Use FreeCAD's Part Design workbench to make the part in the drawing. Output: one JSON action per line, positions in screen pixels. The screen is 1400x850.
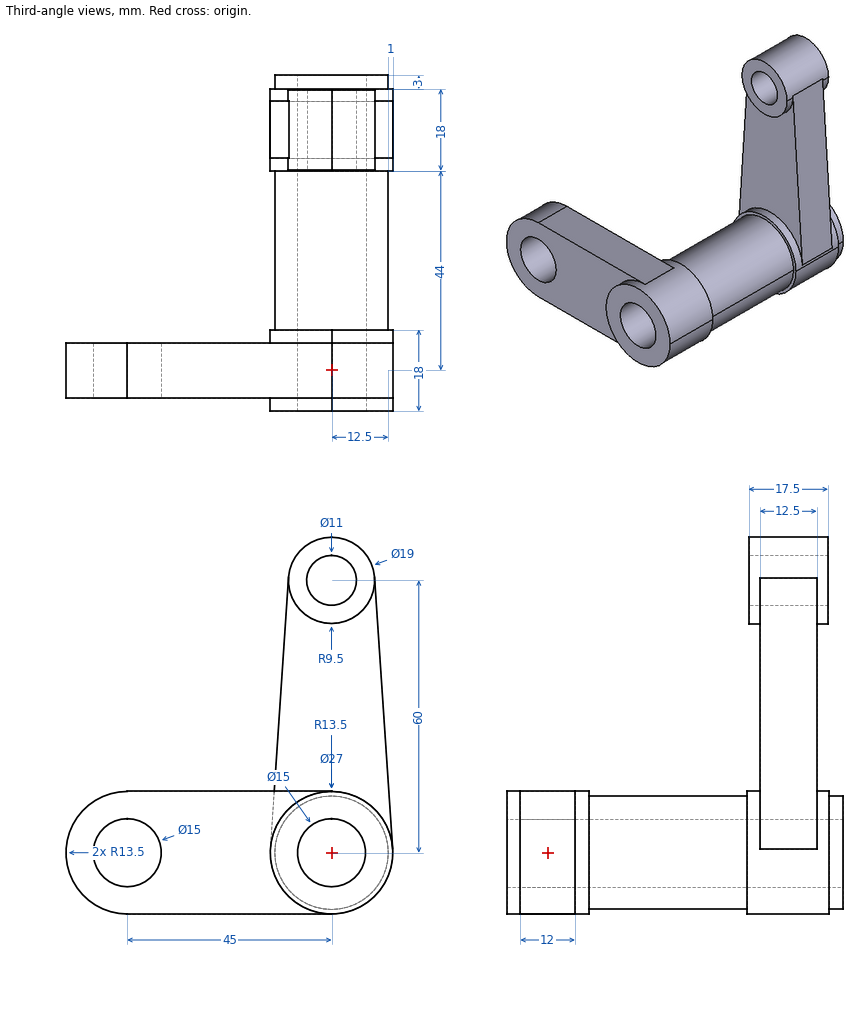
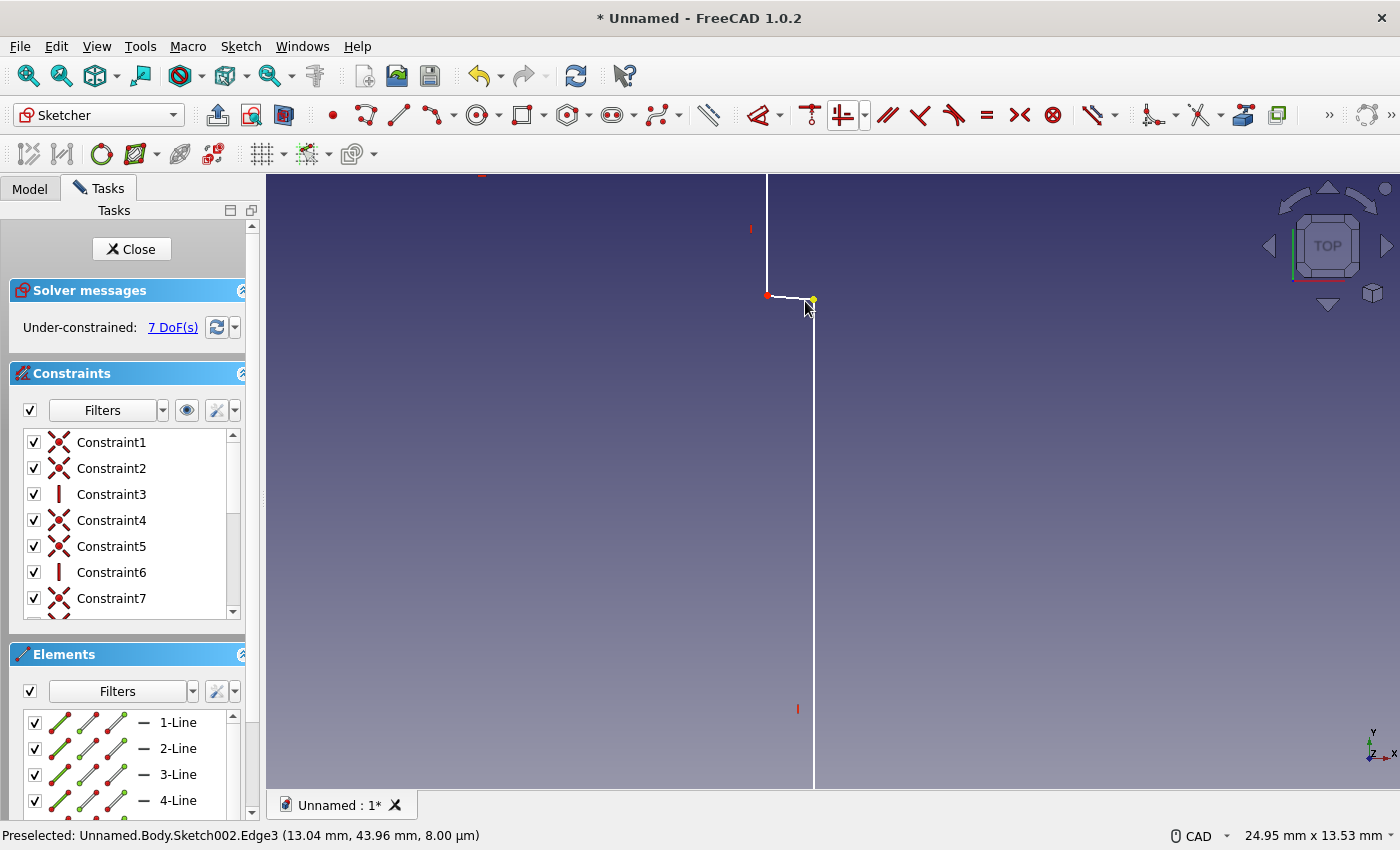
{"action": "left_click", "coordinate": [800, 299]}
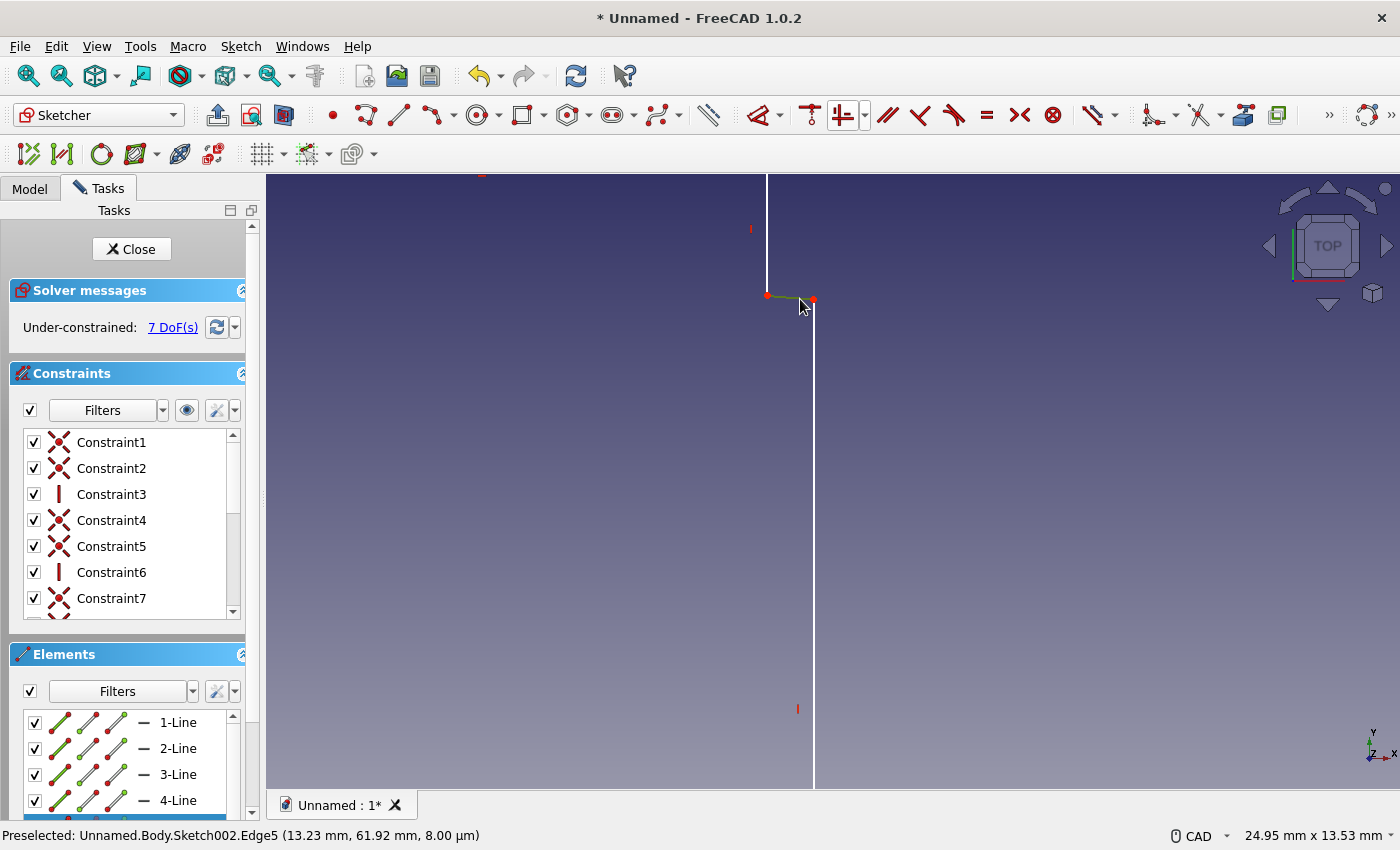
{"action": "key", "text": "h"}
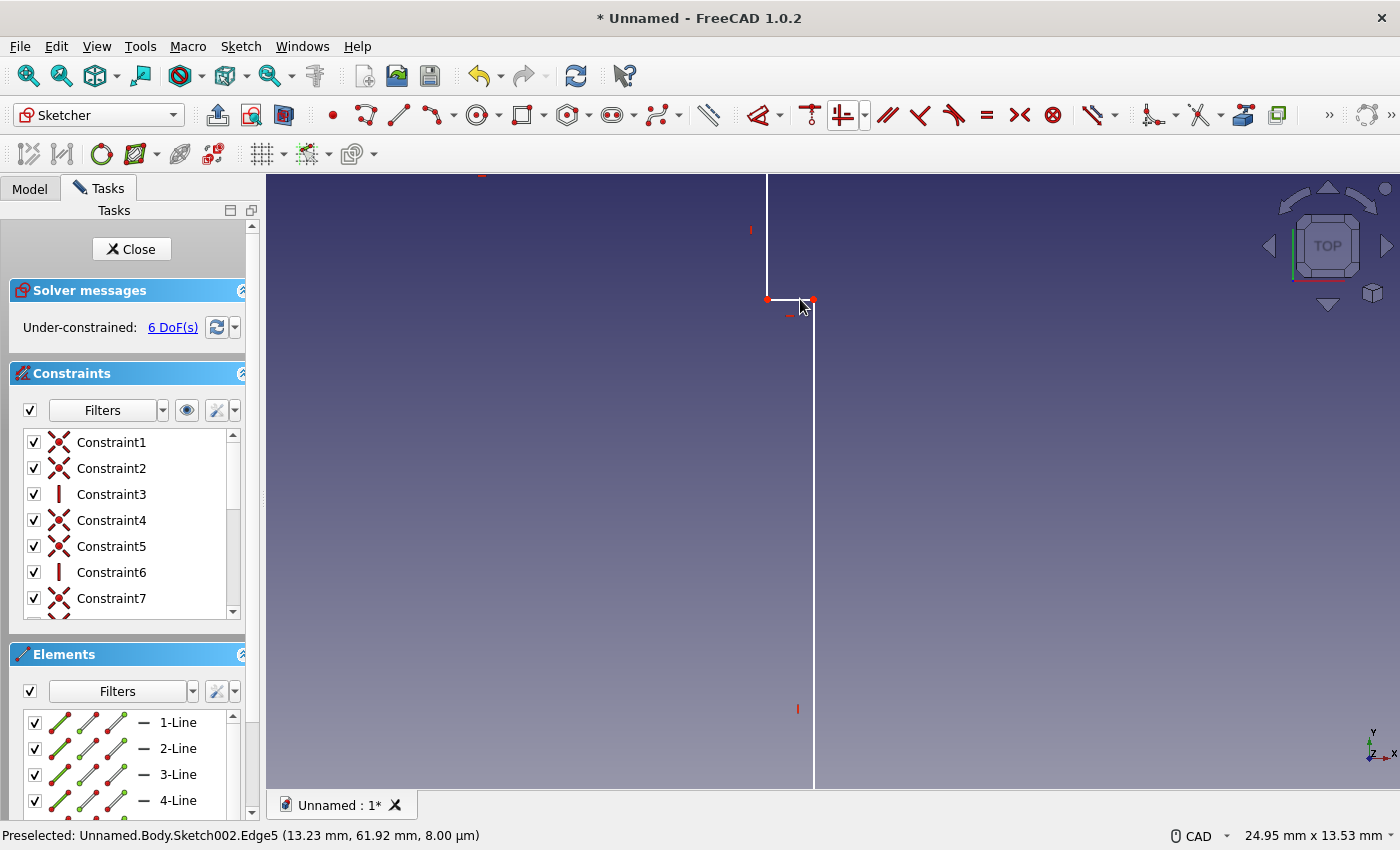
{"action": "key", "text": "d"}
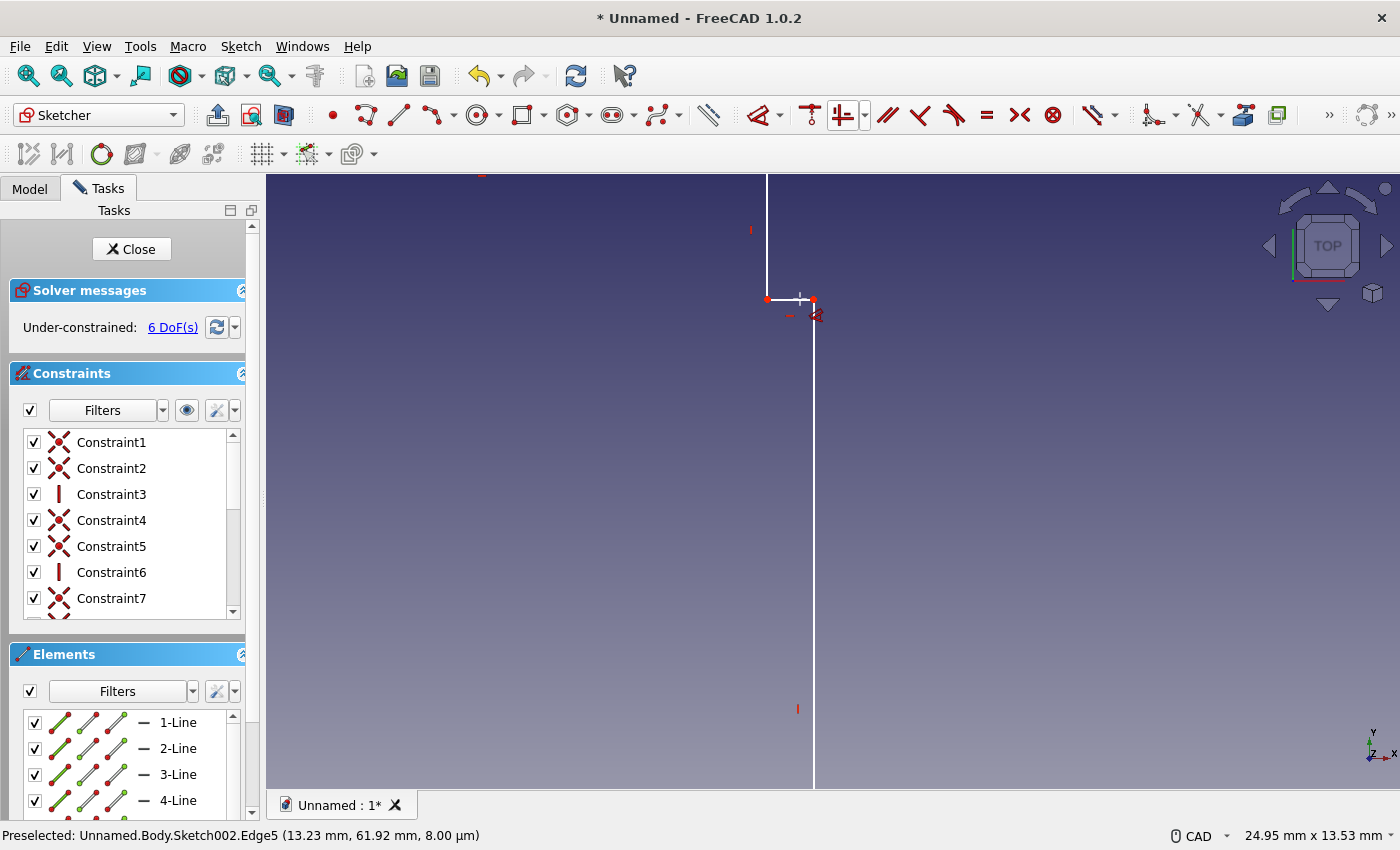
{"action": "scroll", "coordinate": [805, 301], "scroll_direction": "down", "scroll_amount": 10}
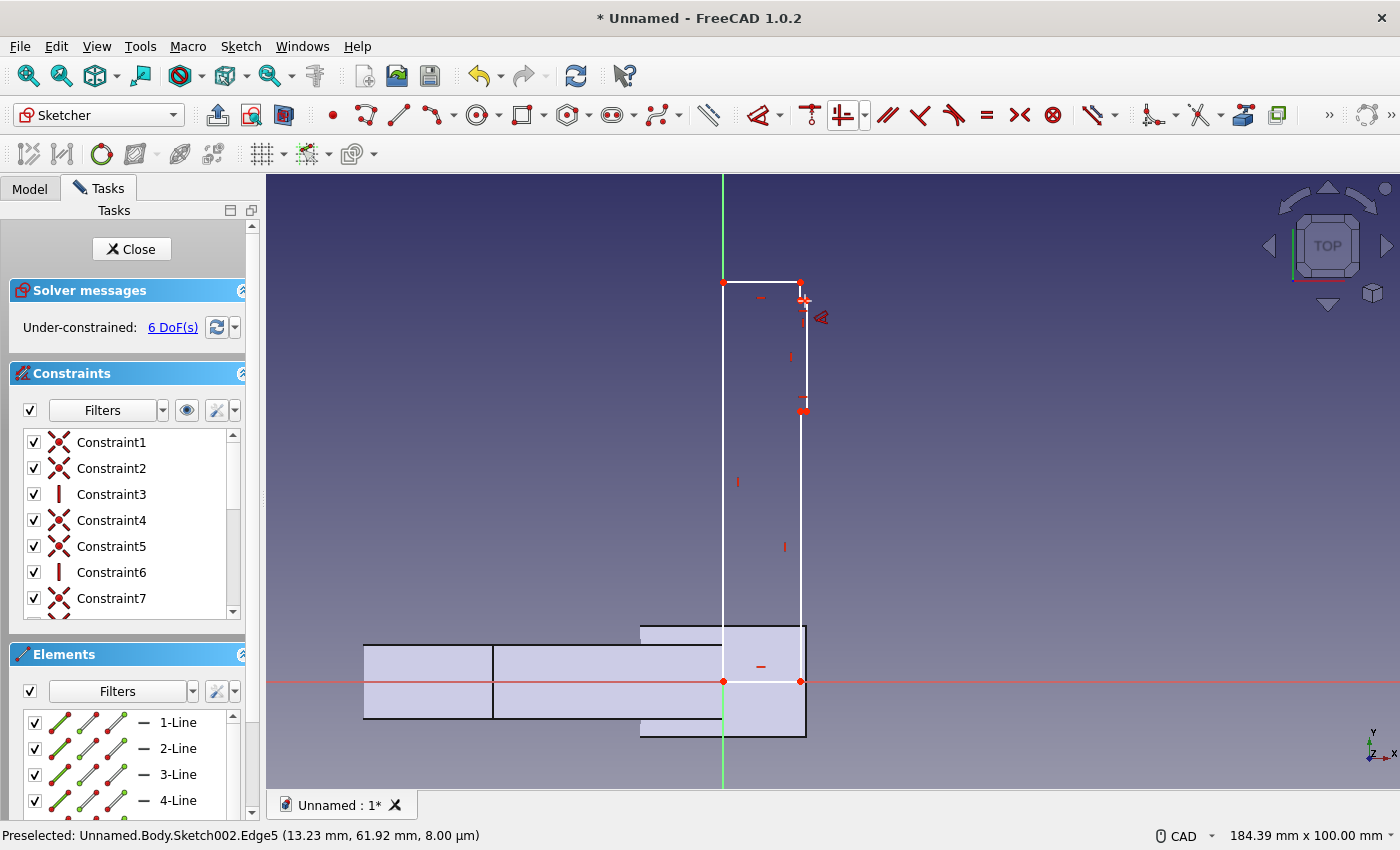
{"action": "scroll", "coordinate": [802, 412], "scroll_direction": "up", "scroll_amount": 11}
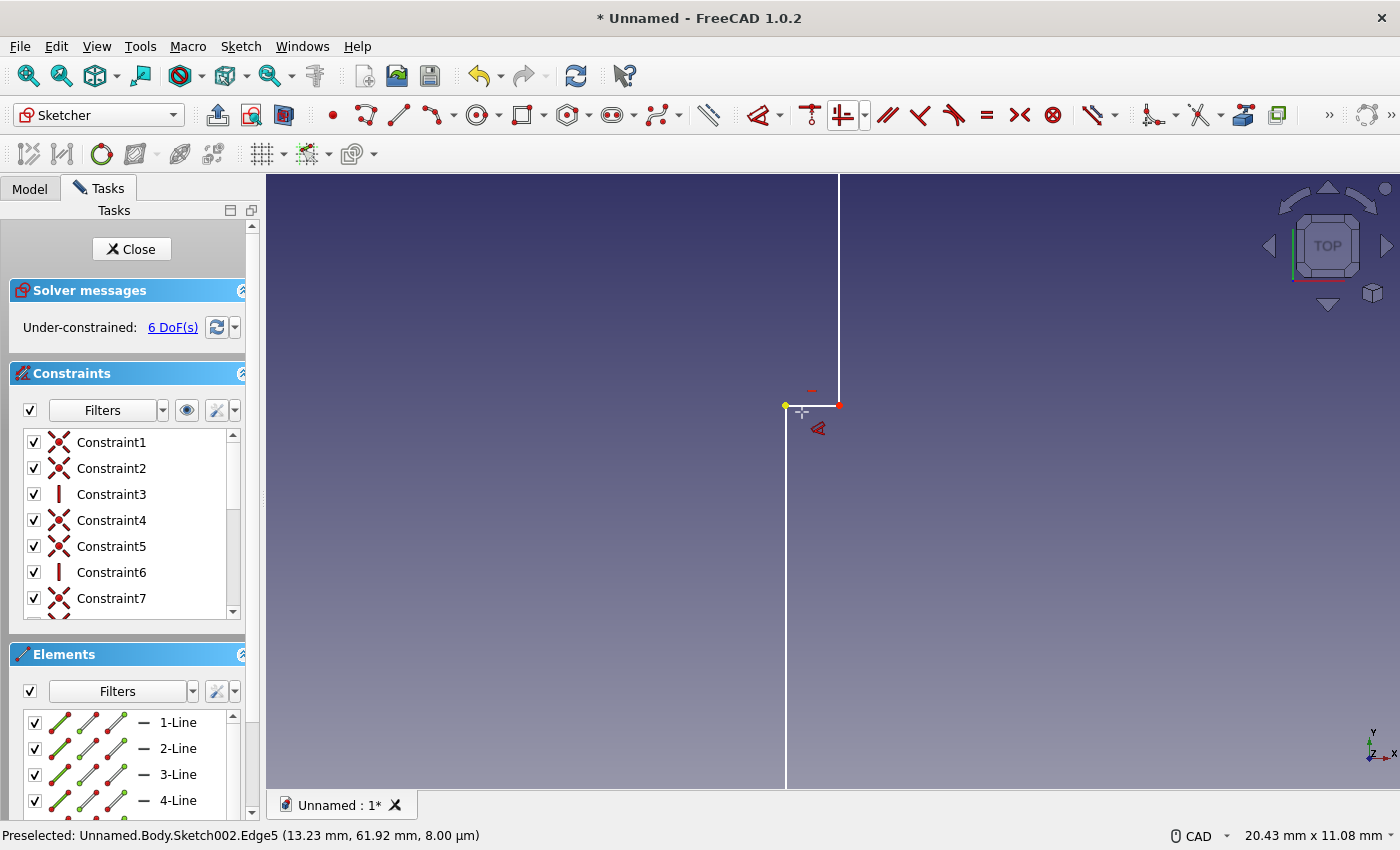
{"action": "left_click", "coordinate": [802, 406]}
{"action": "left_click", "coordinate": [813, 372]}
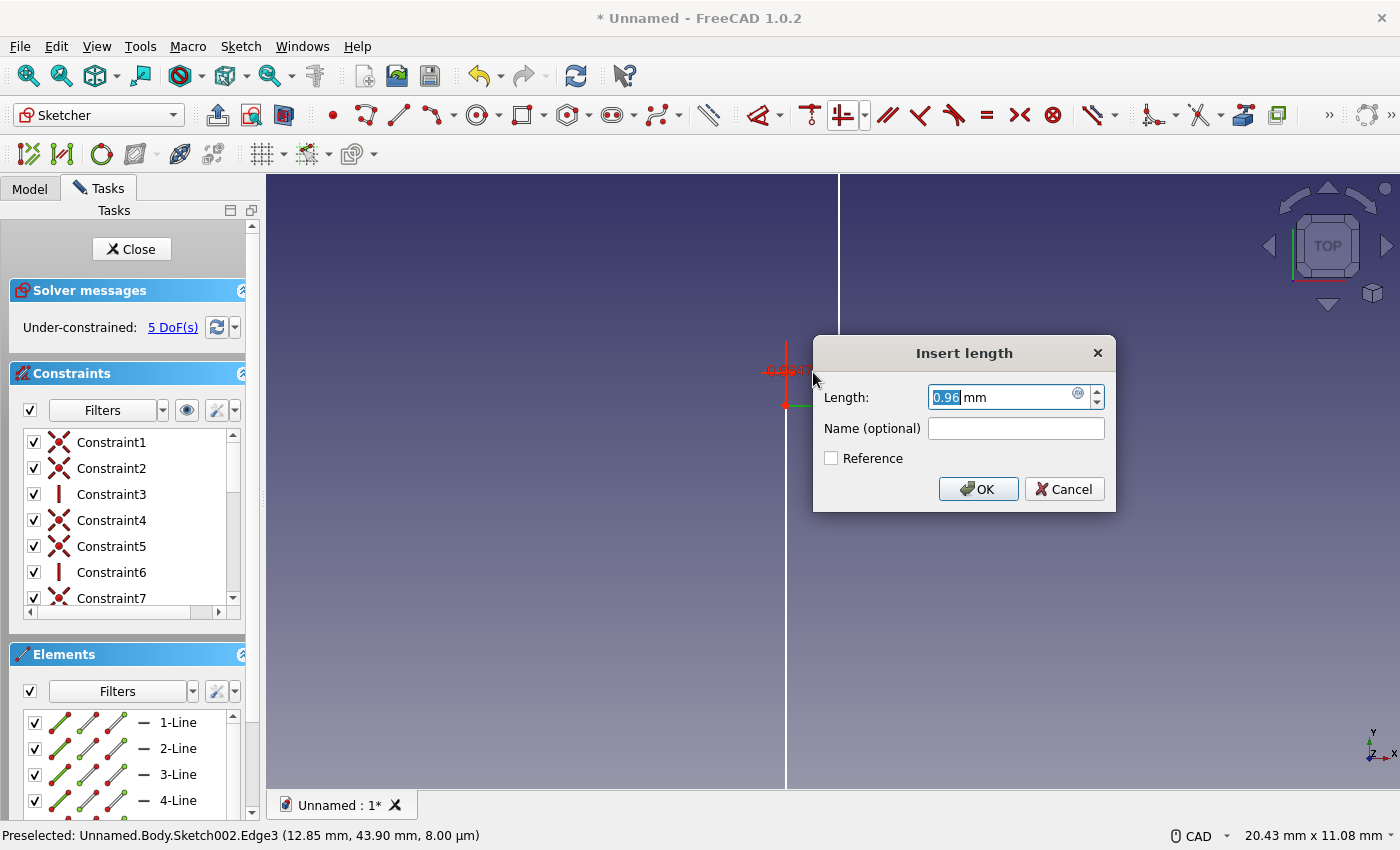
{"action": "type", "text": "1"}
{"action": "key", "text": "Return"}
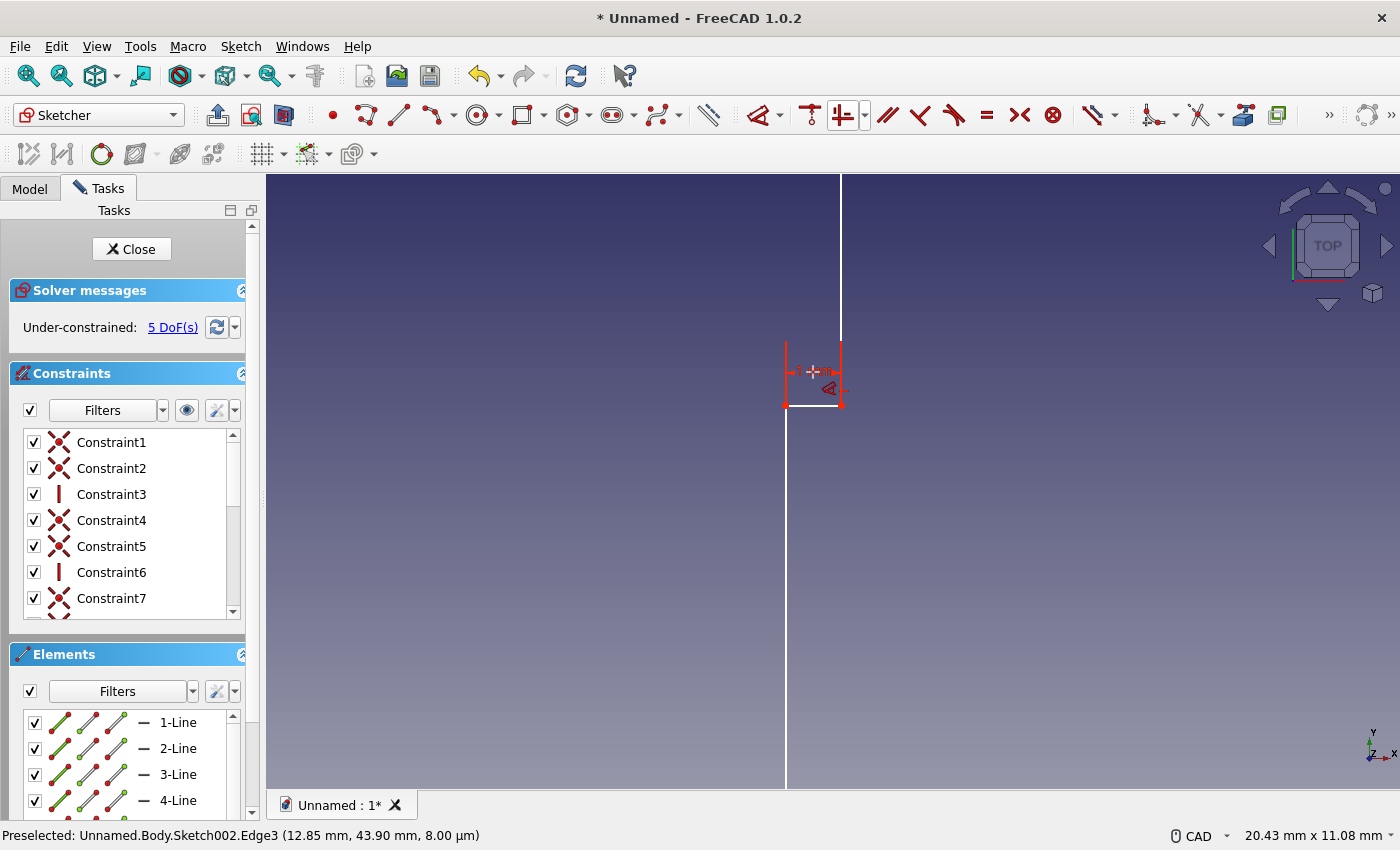
{"action": "scroll", "coordinate": [802, 412], "scroll_direction": "down", "scroll_amount": 11}